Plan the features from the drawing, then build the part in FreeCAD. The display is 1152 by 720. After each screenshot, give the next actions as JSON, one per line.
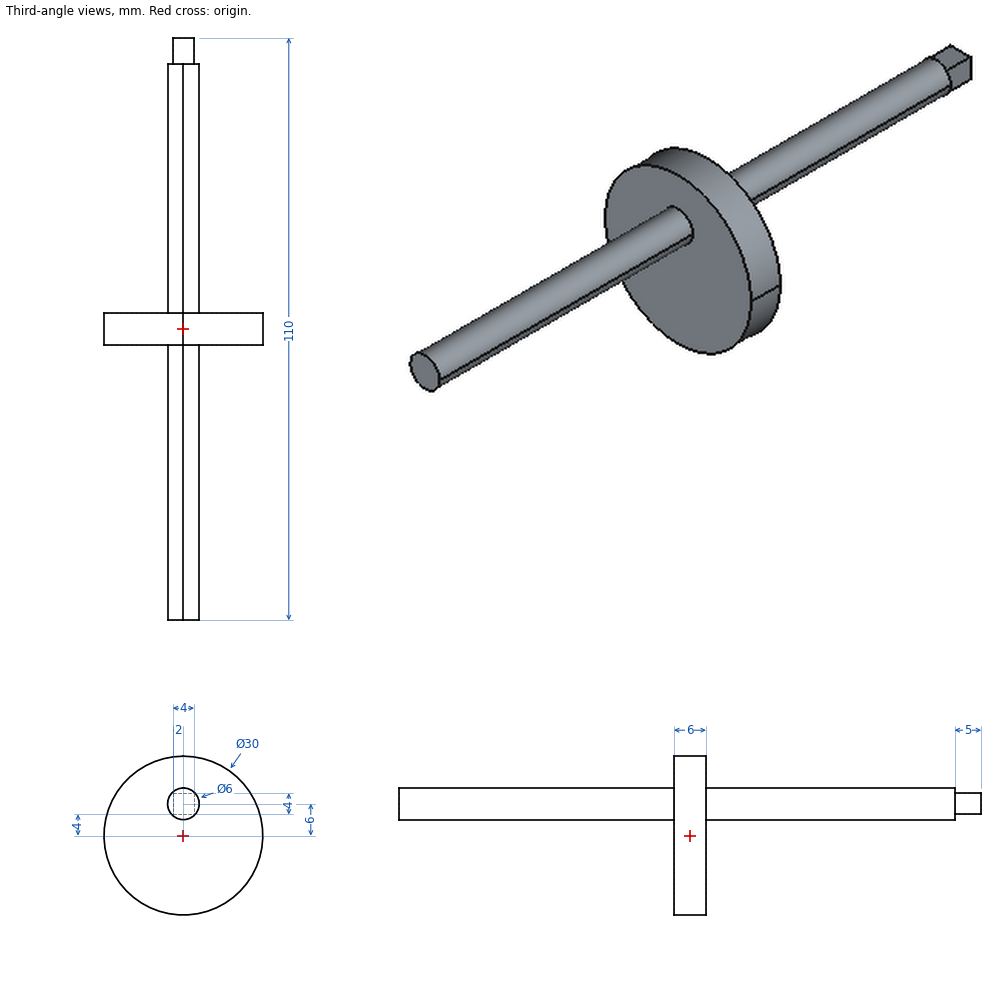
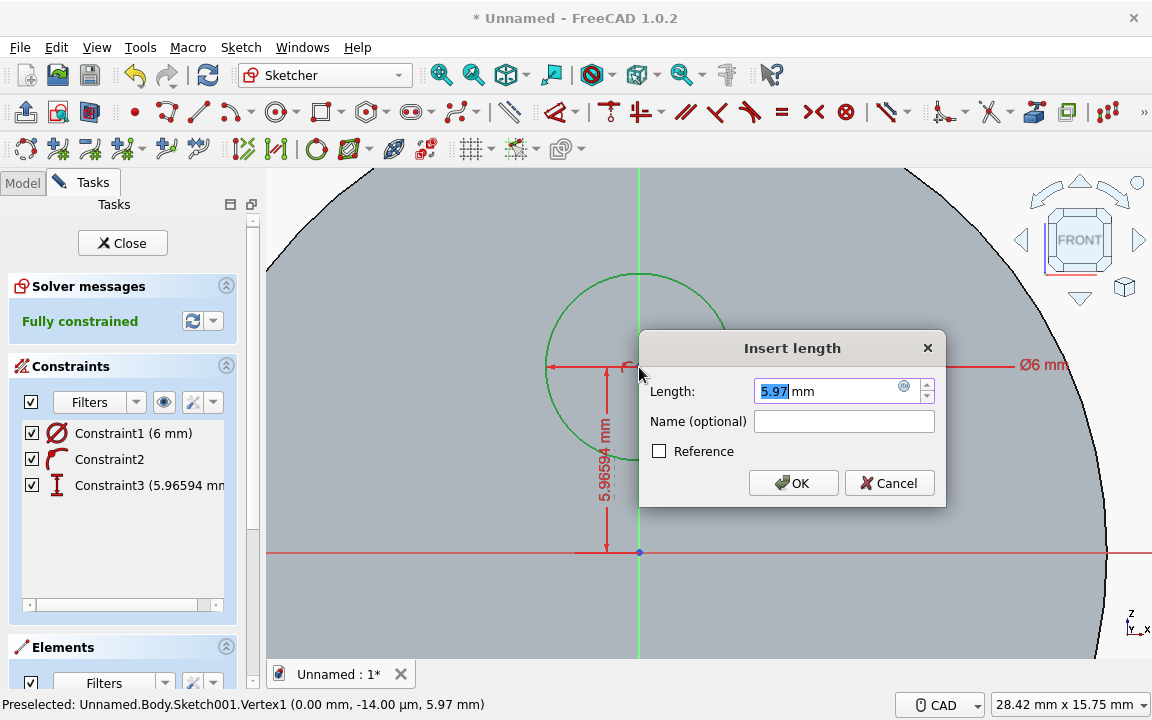
{"action": "type", "text": "6"}
{"action": "key", "text": "Return"}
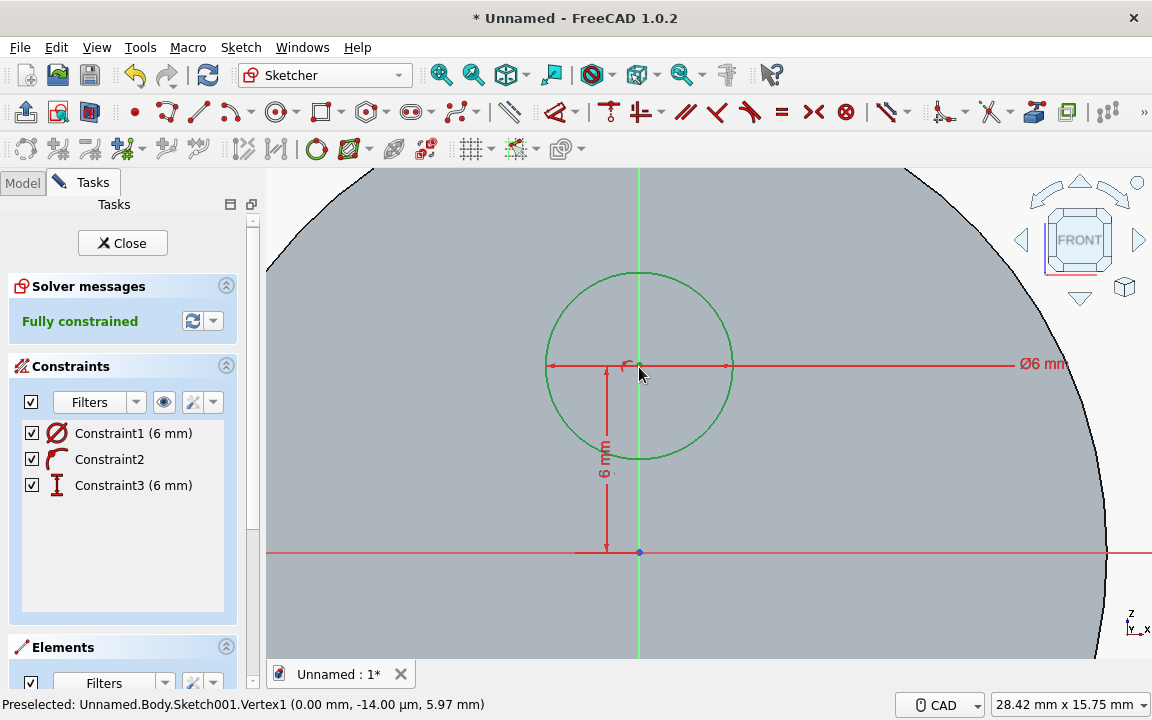
{"action": "left_click", "coordinate": [123, 243]}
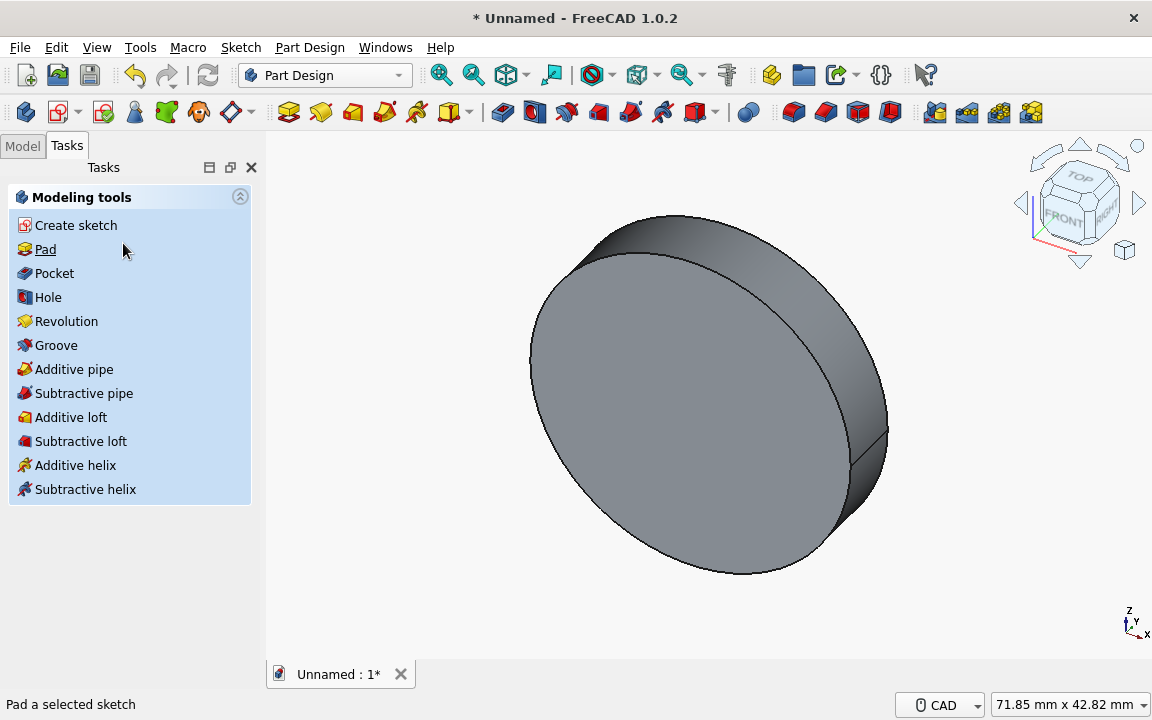
{"action": "left_click", "coordinate": [290, 112]}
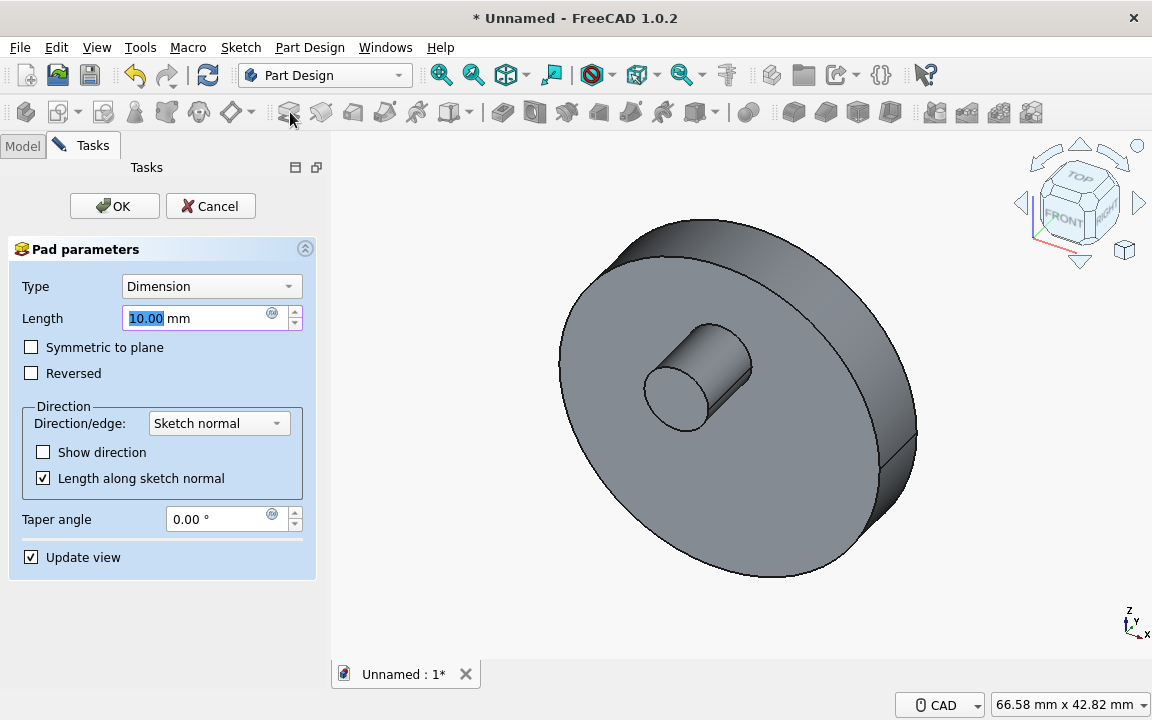
{"action": "type", "text": "110"}
{"action": "key", "text": "Tab"}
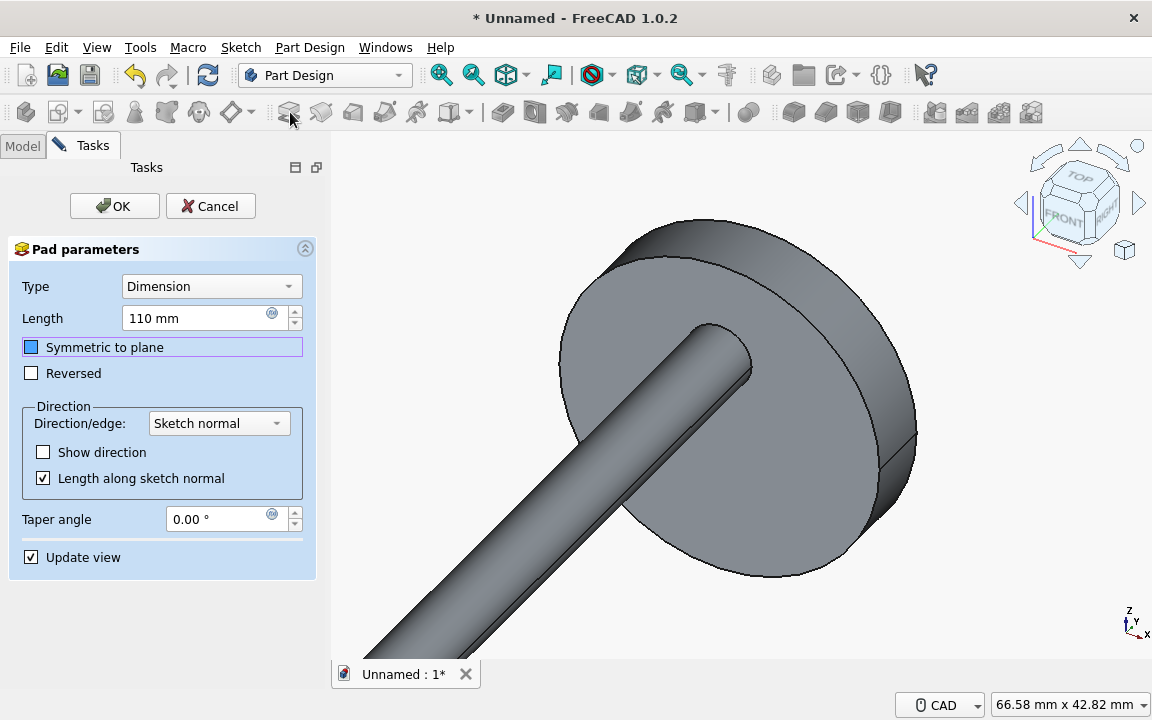
{"action": "left_click", "coordinate": [30, 347]}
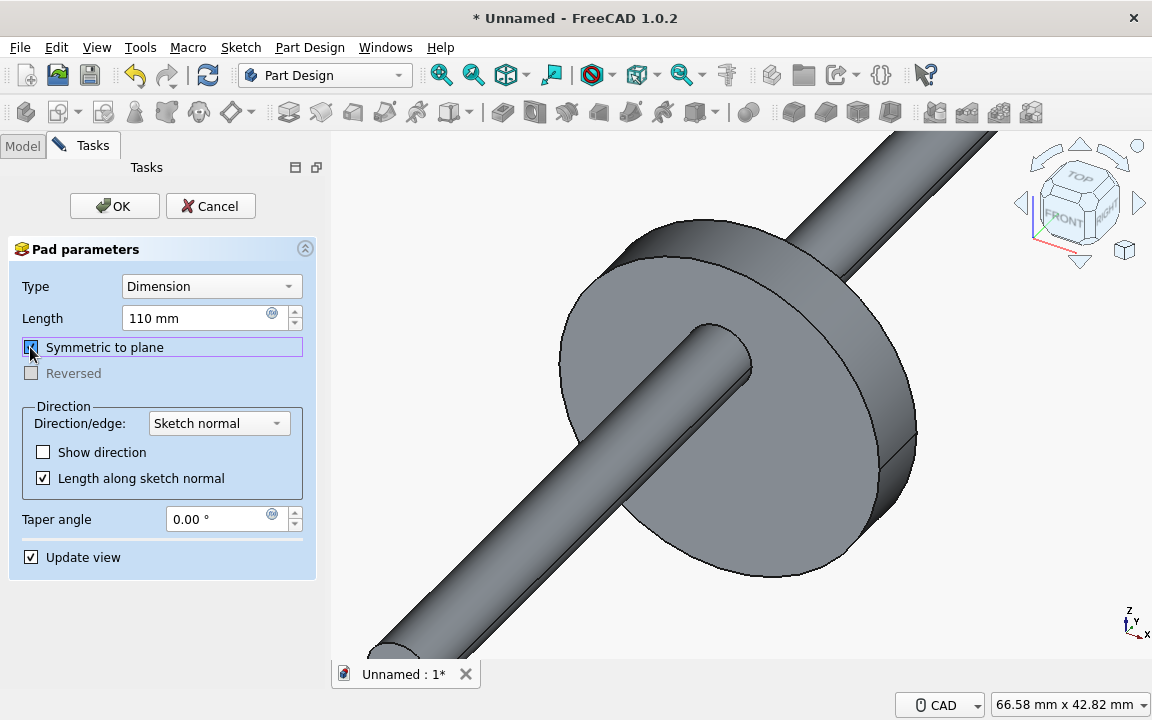
{"action": "left_click", "coordinate": [115, 206]}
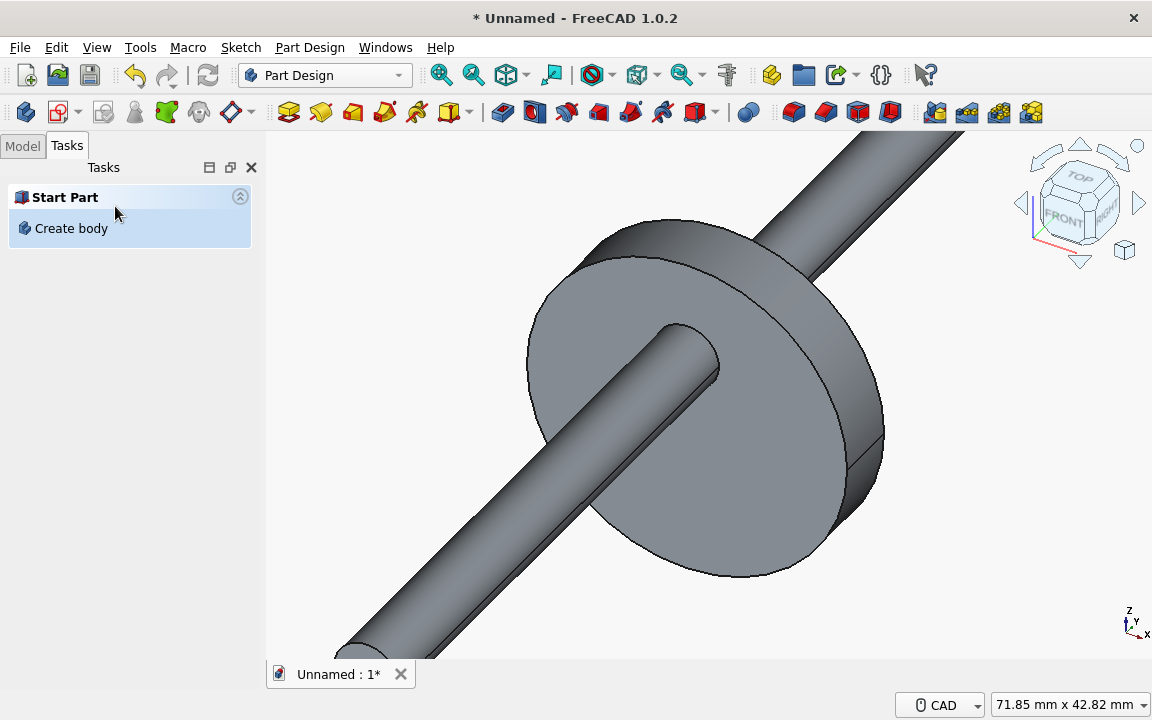
{"action": "key", "text": "v f"}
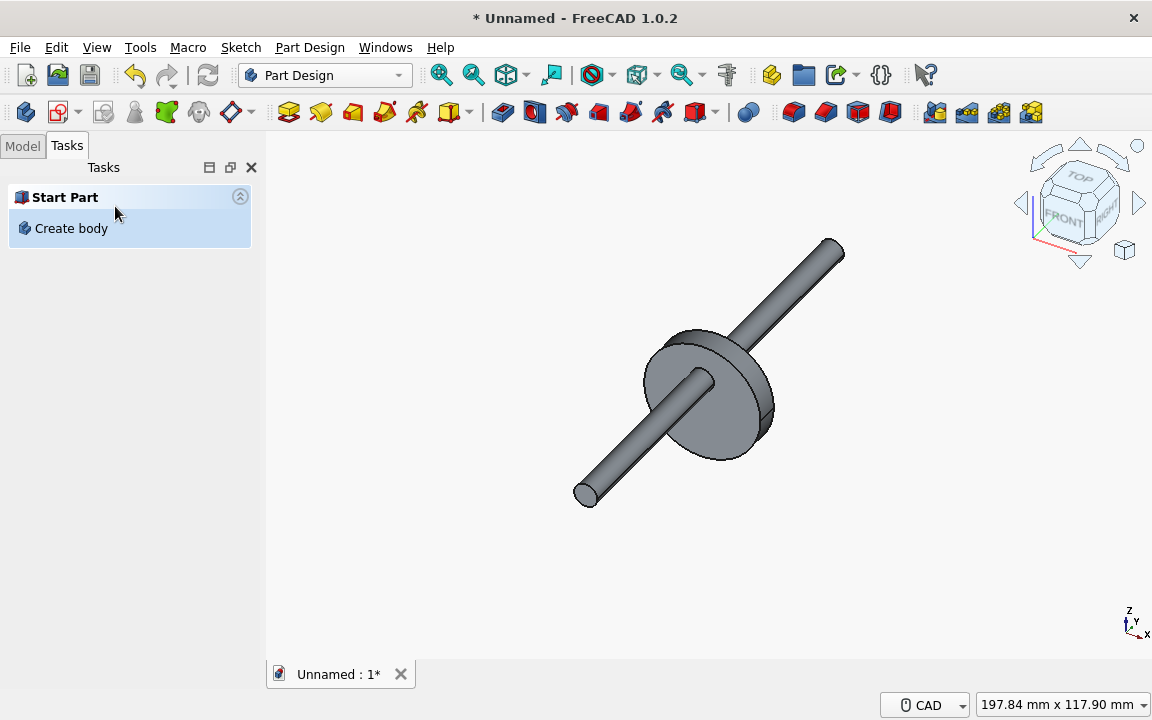
{"action": "key", "text": "4"}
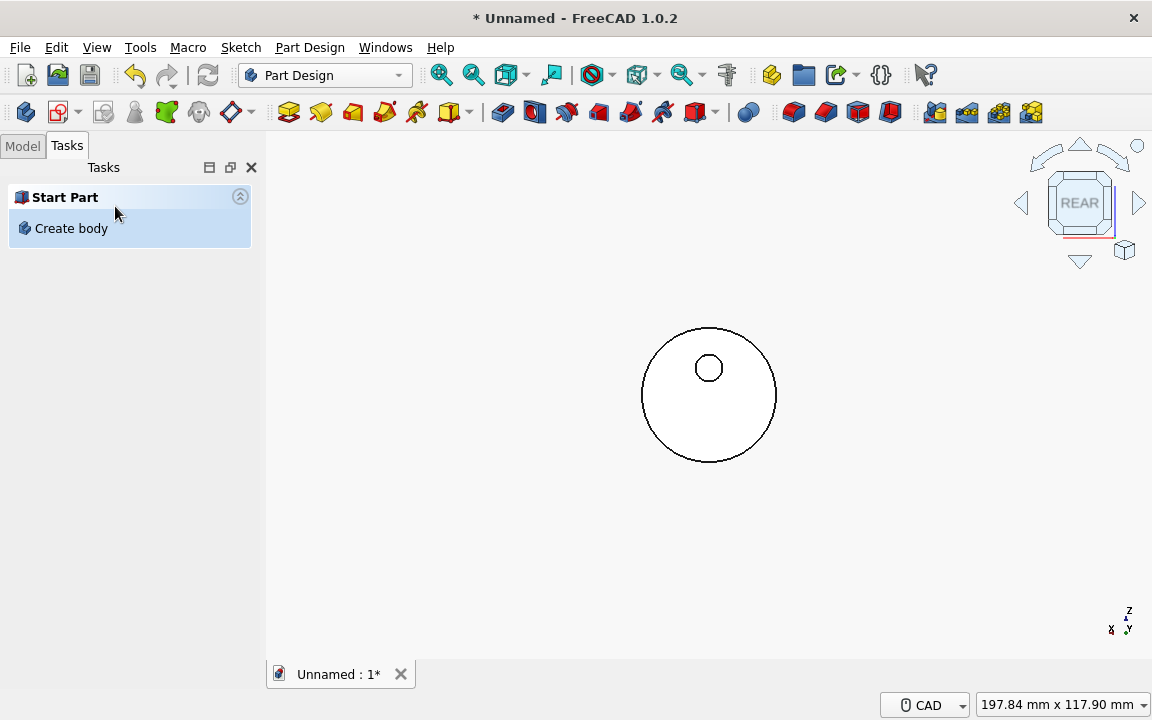
{"action": "key", "text": "v f"}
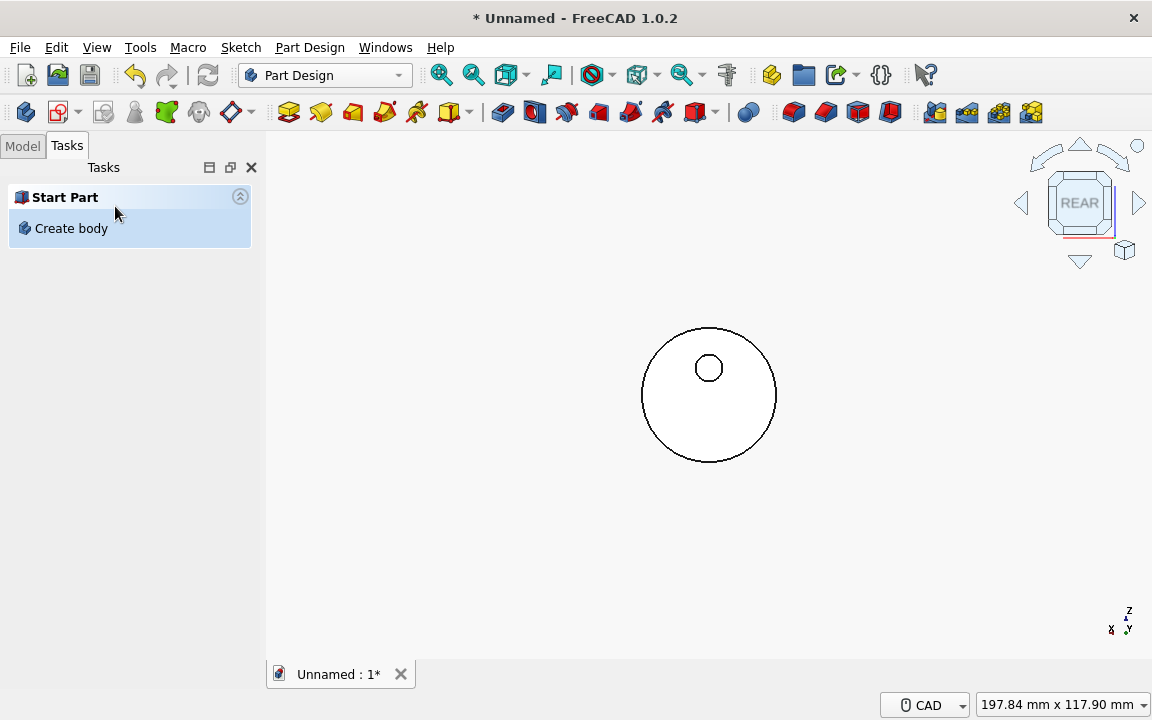
{"action": "left_click", "coordinate": [709, 367]}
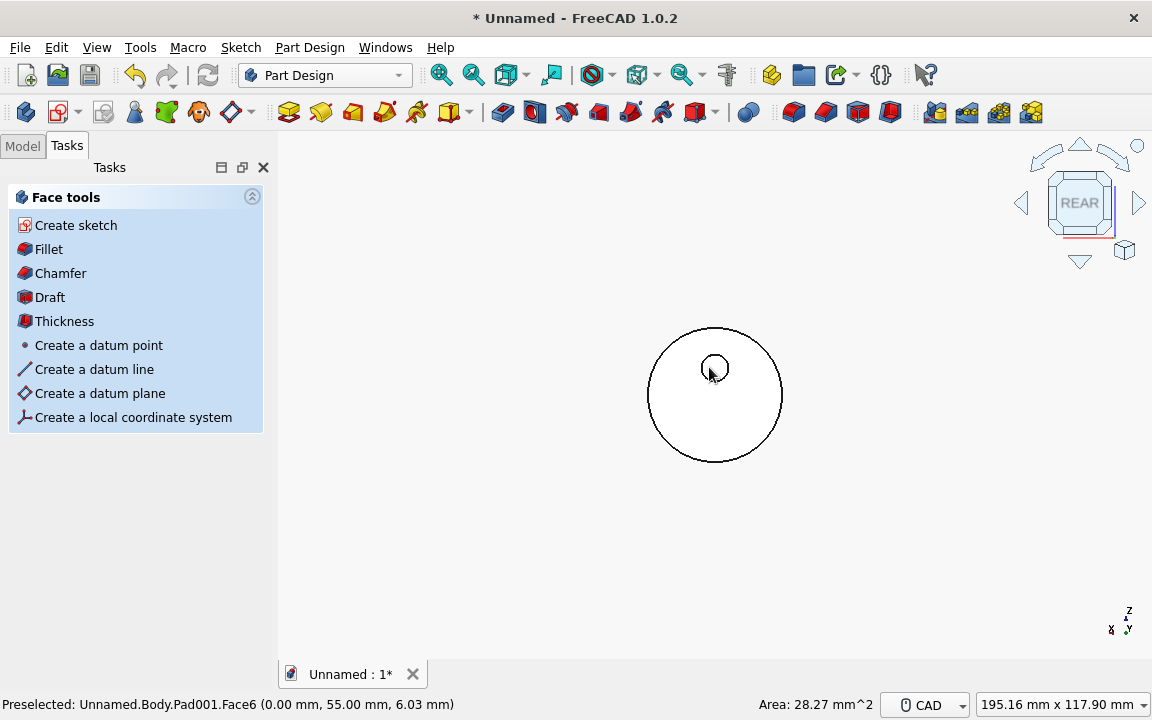
{"action": "left_click", "coordinate": [58, 112]}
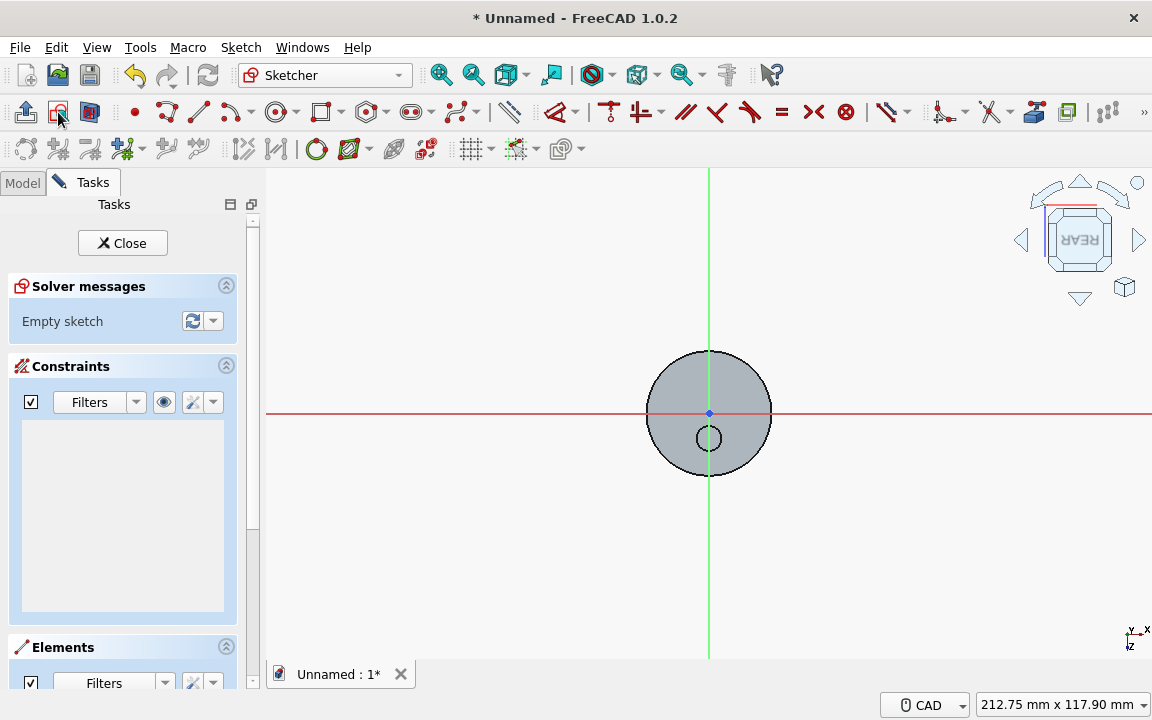
{"action": "scroll", "coordinate": [718, 435], "scroll_direction": "up", "scroll_amount": 11}